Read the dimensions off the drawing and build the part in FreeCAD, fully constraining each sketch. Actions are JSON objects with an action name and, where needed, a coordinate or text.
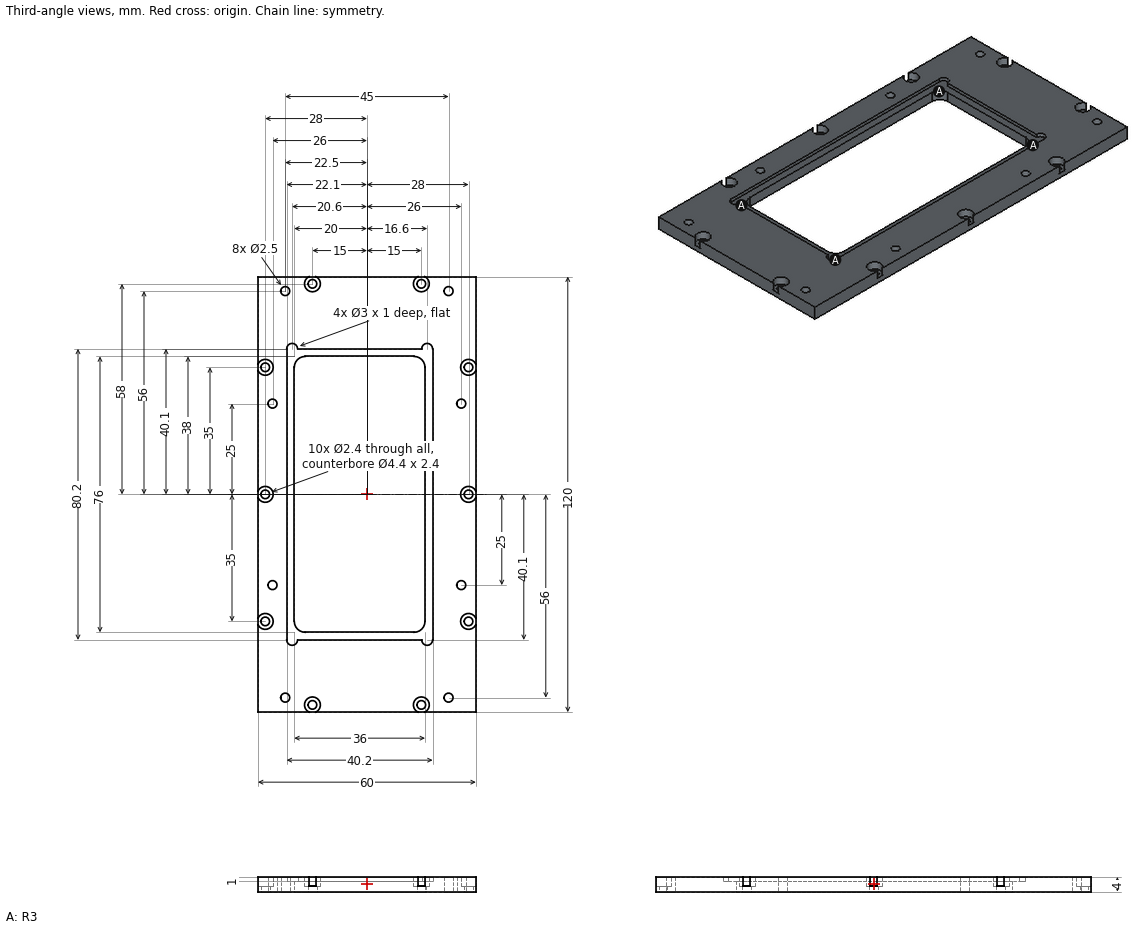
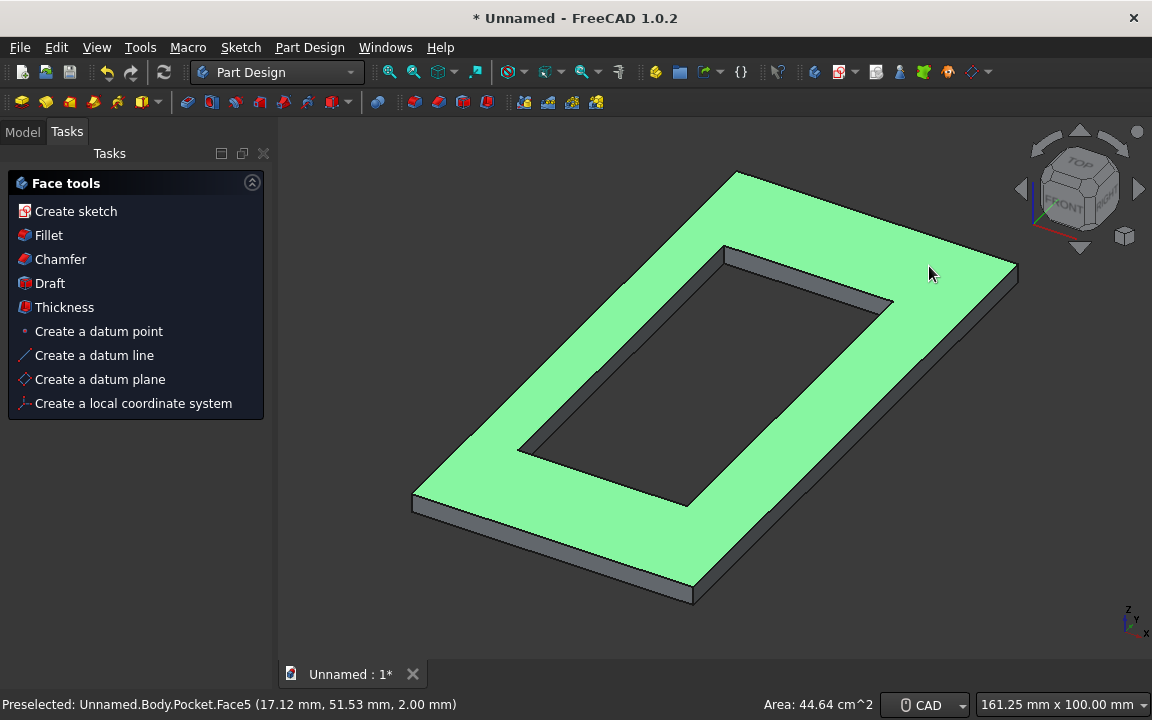
{"action": "left_click", "coordinate": [840, 72]}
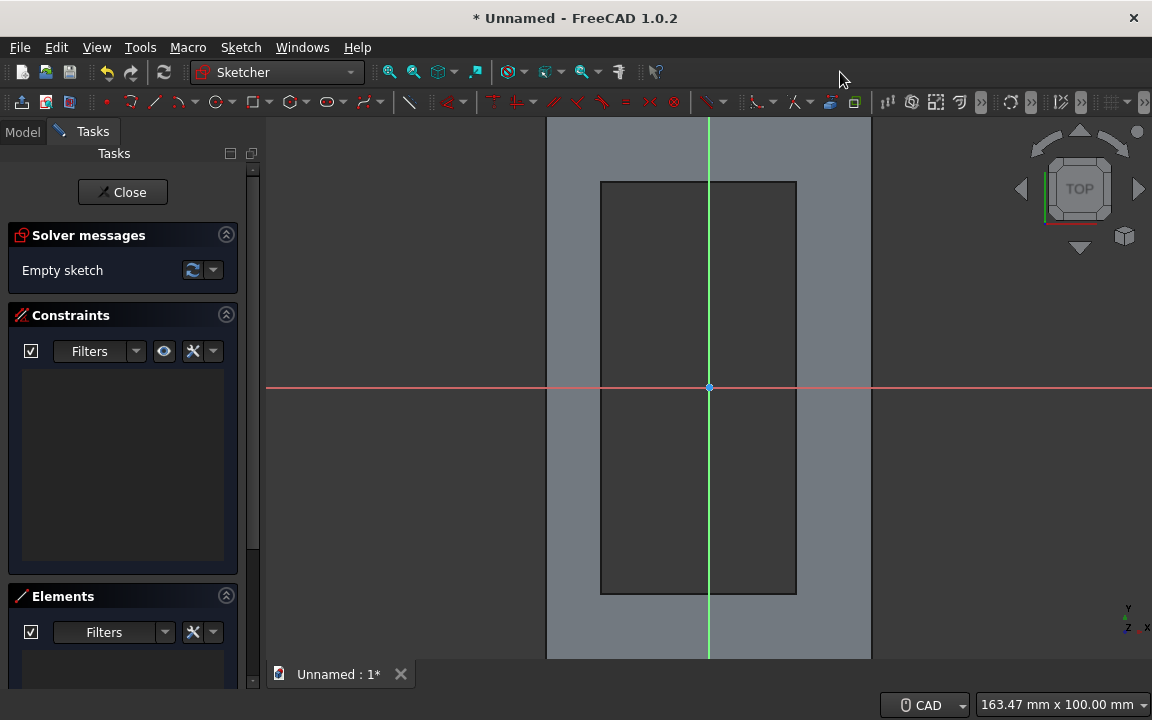
{"action": "key", "text": "g r"}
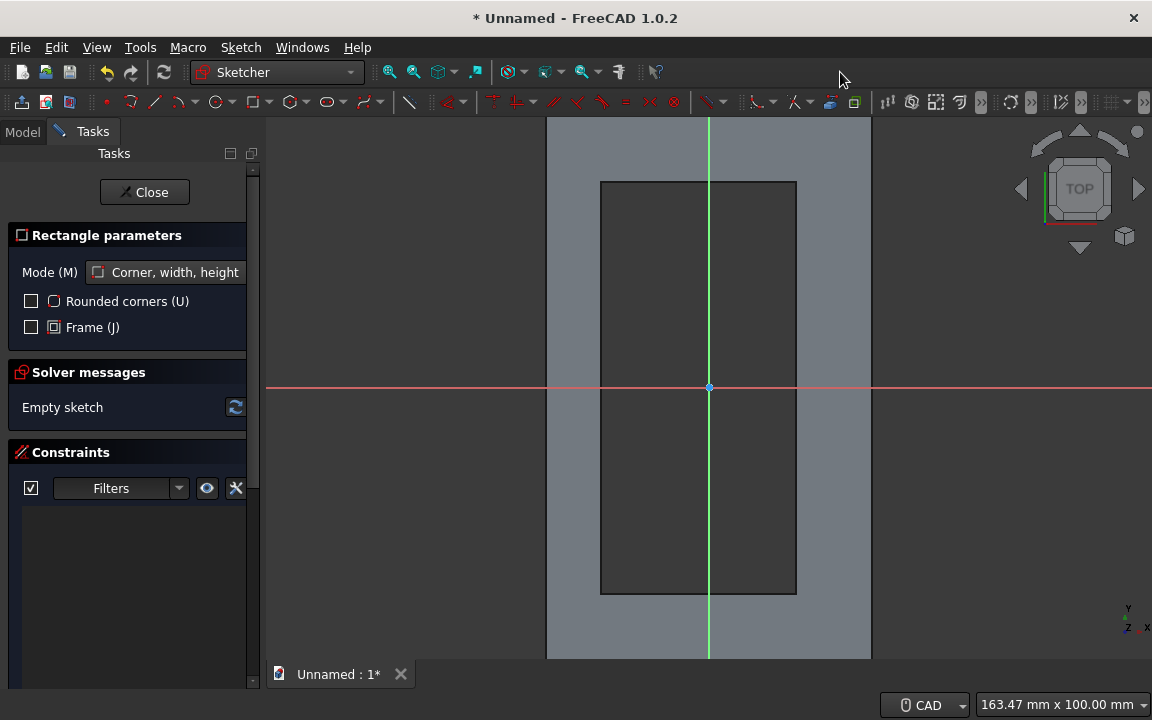
{"action": "left_click", "coordinate": [589, 171]}
{"action": "left_click", "coordinate": [807, 605]}
{"action": "key", "text": "Escape"}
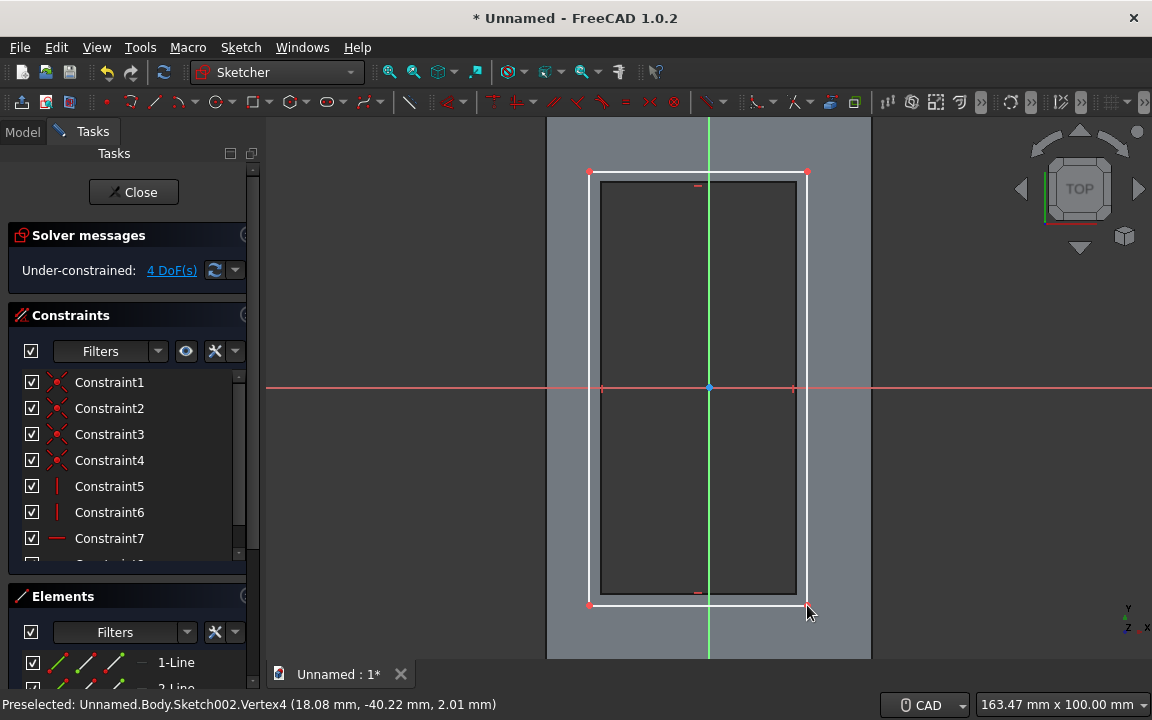
{"action": "left_click", "coordinate": [448, 102]}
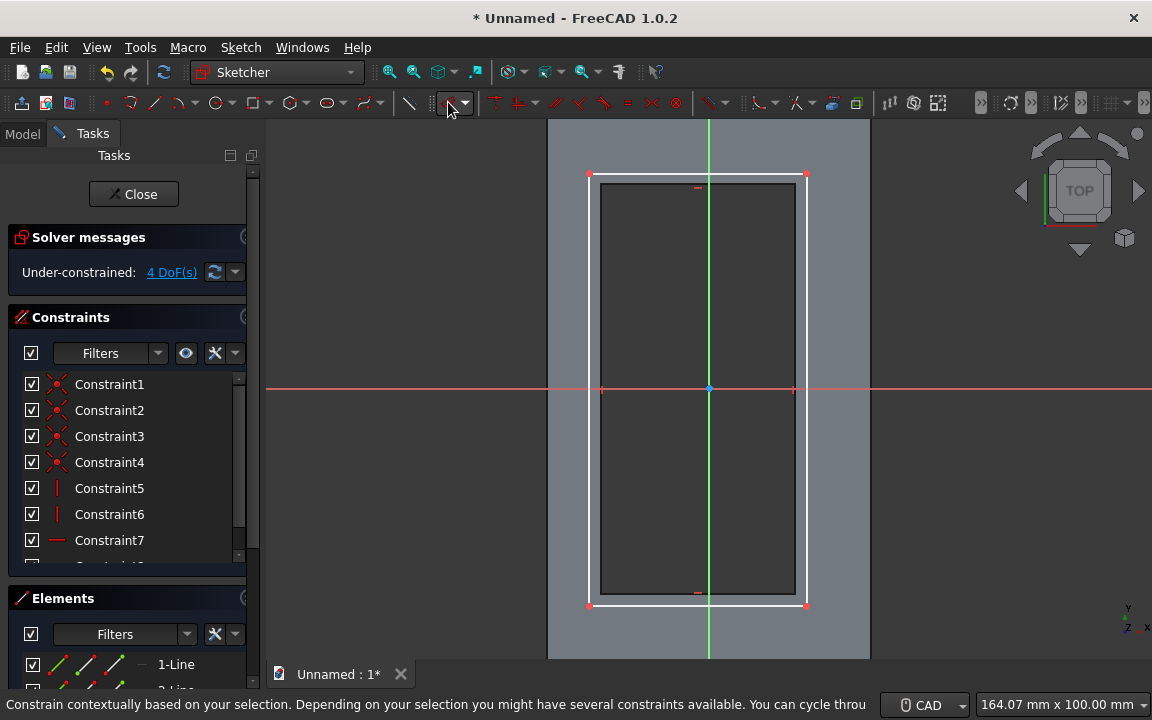
{"action": "left_click", "coordinate": [589, 304]}
{"action": "left_click", "coordinate": [555, 291]}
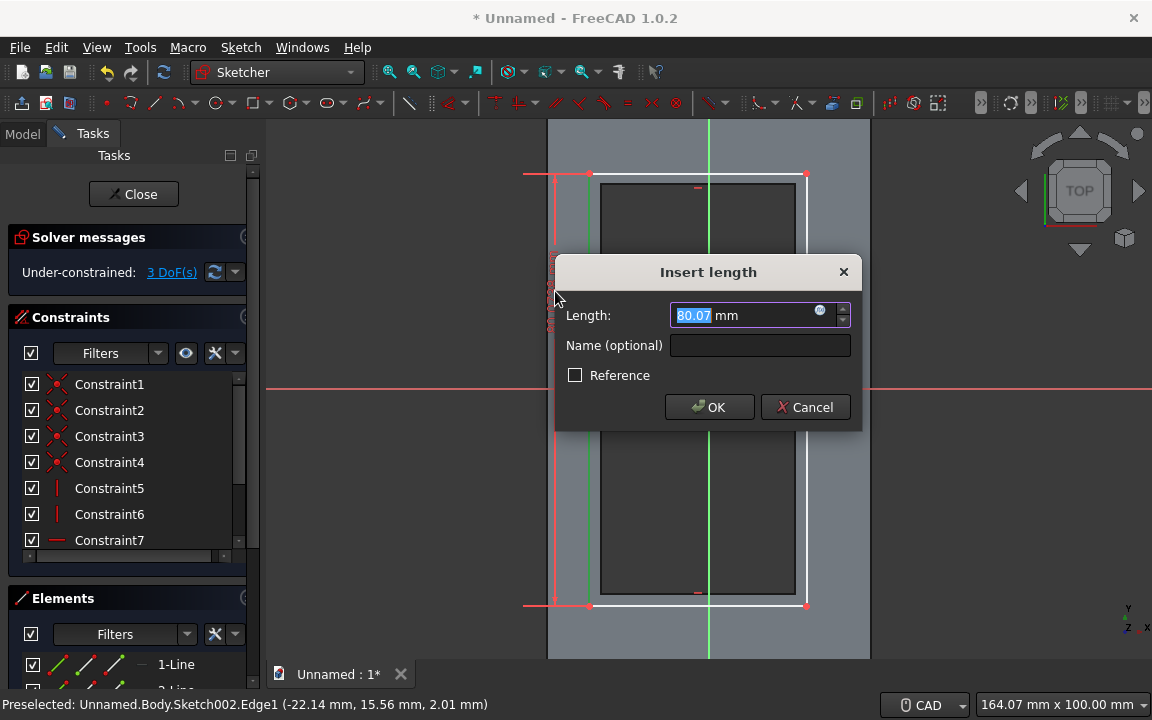
{"action": "type", "text": "80.2"}
{"action": "key", "text": "Return"}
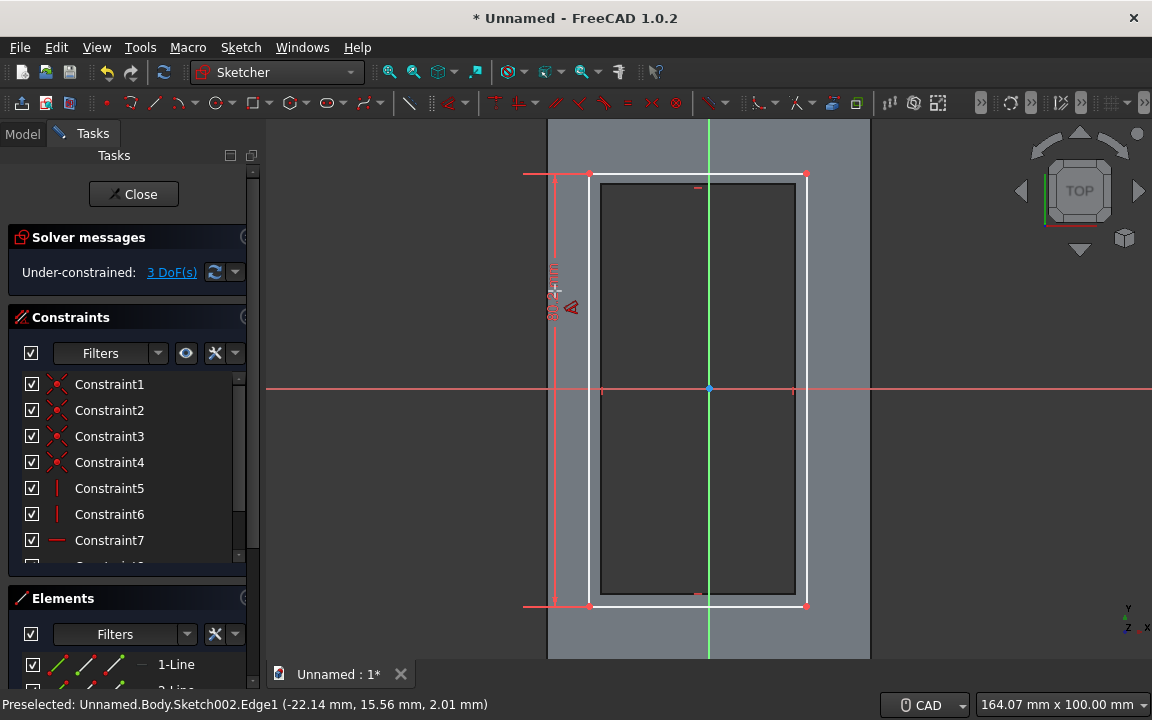
{"action": "left_click", "coordinate": [655, 607]}
{"action": "left_click", "coordinate": [648, 573]}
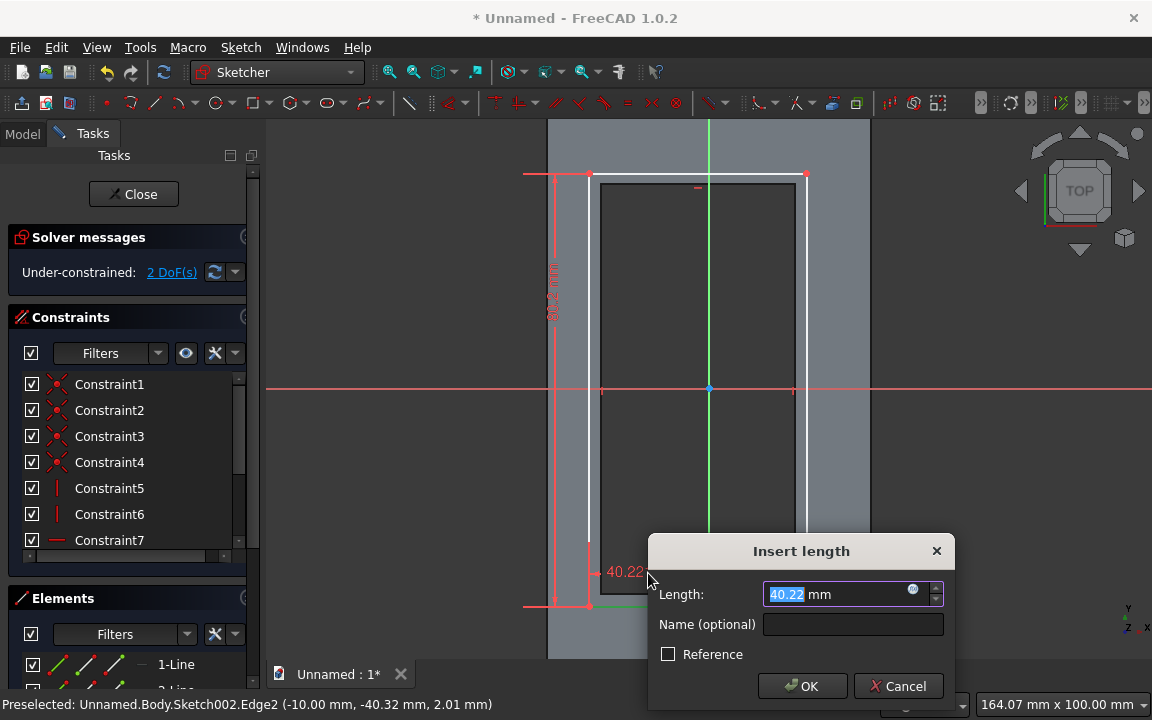
{"action": "type", "text": "40.2"}
{"action": "key", "text": "Return"}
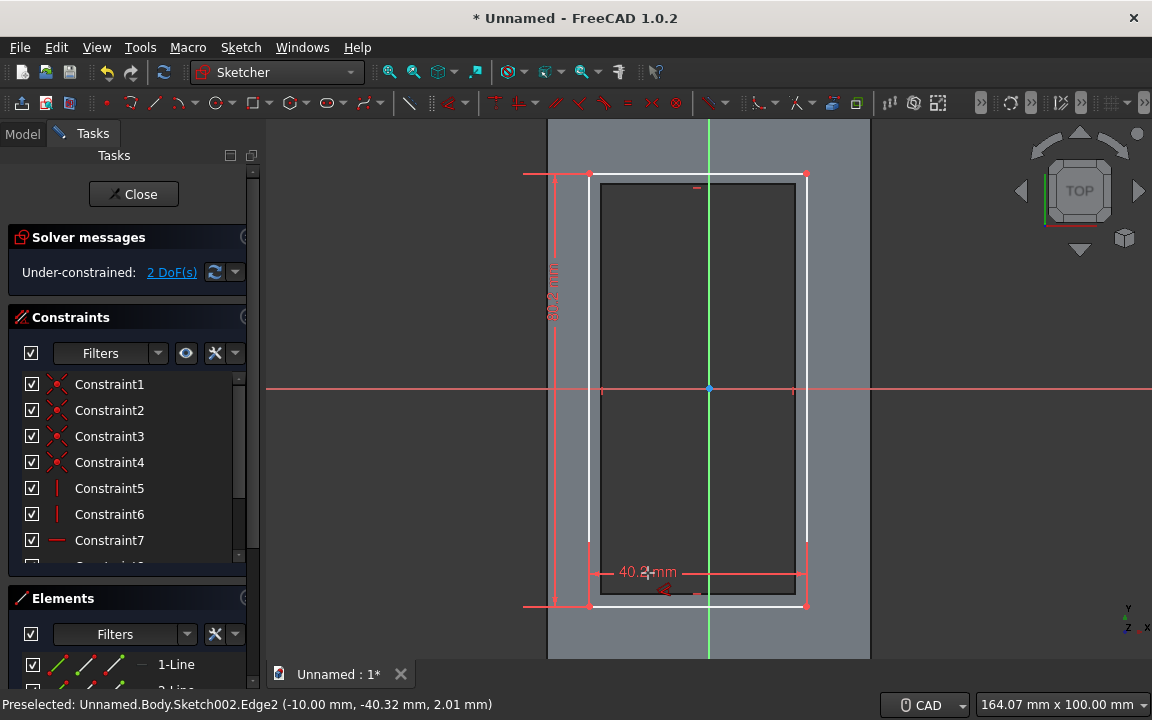
{"action": "left_click", "coordinate": [589, 174]}
{"action": "left_click", "coordinate": [649, 423]}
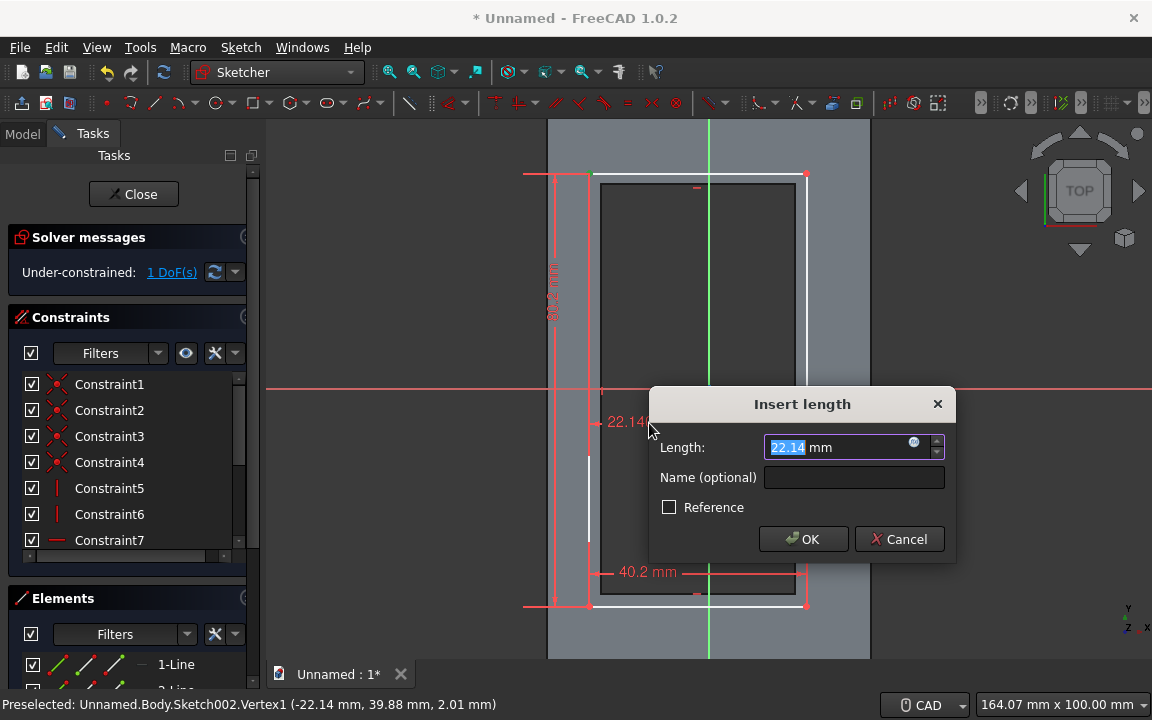
{"action": "type", "text": "22.1"}
{"action": "key", "text": "Return"}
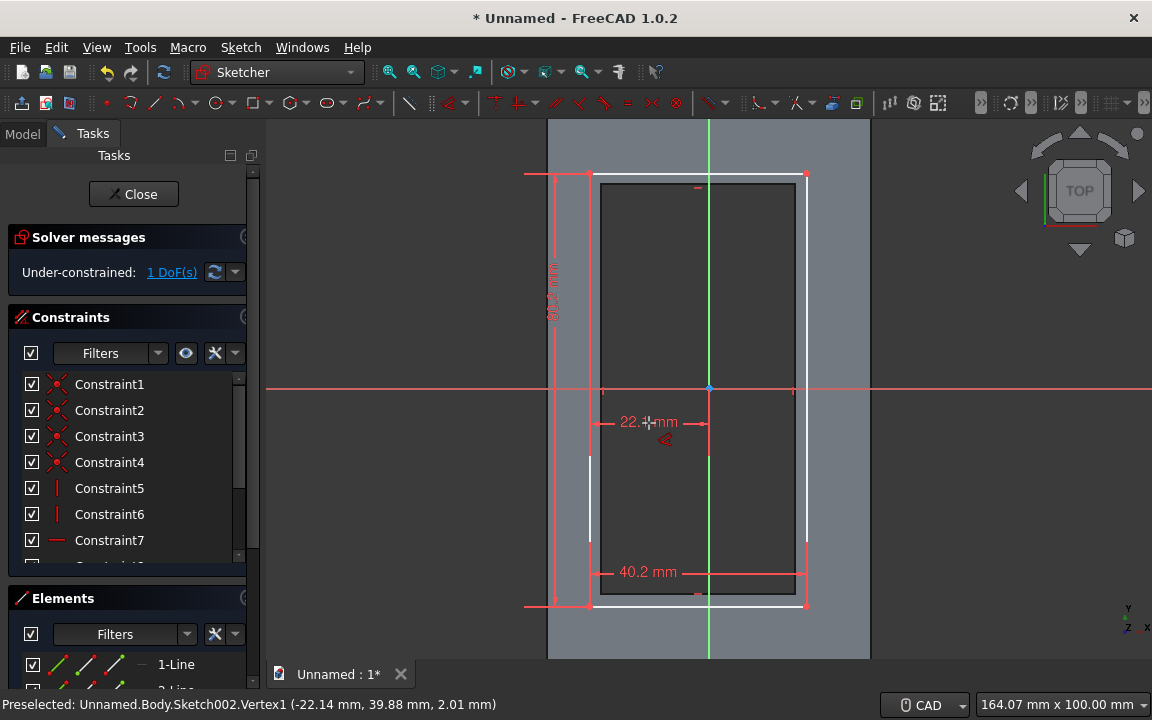
{"action": "left_click", "coordinate": [590, 174]}
{"action": "left_click", "coordinate": [556, 232]}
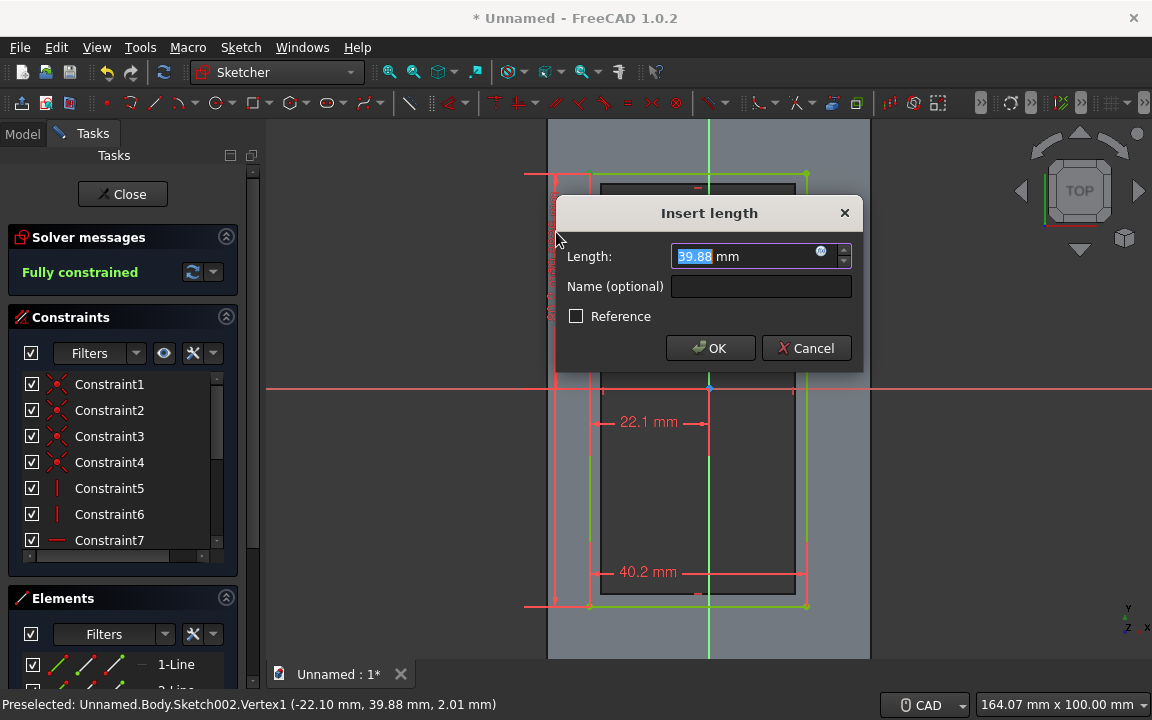
{"action": "type", "text": "40.1"}
{"action": "key", "text": "Return"}
{"action": "key", "text": "Escape"}